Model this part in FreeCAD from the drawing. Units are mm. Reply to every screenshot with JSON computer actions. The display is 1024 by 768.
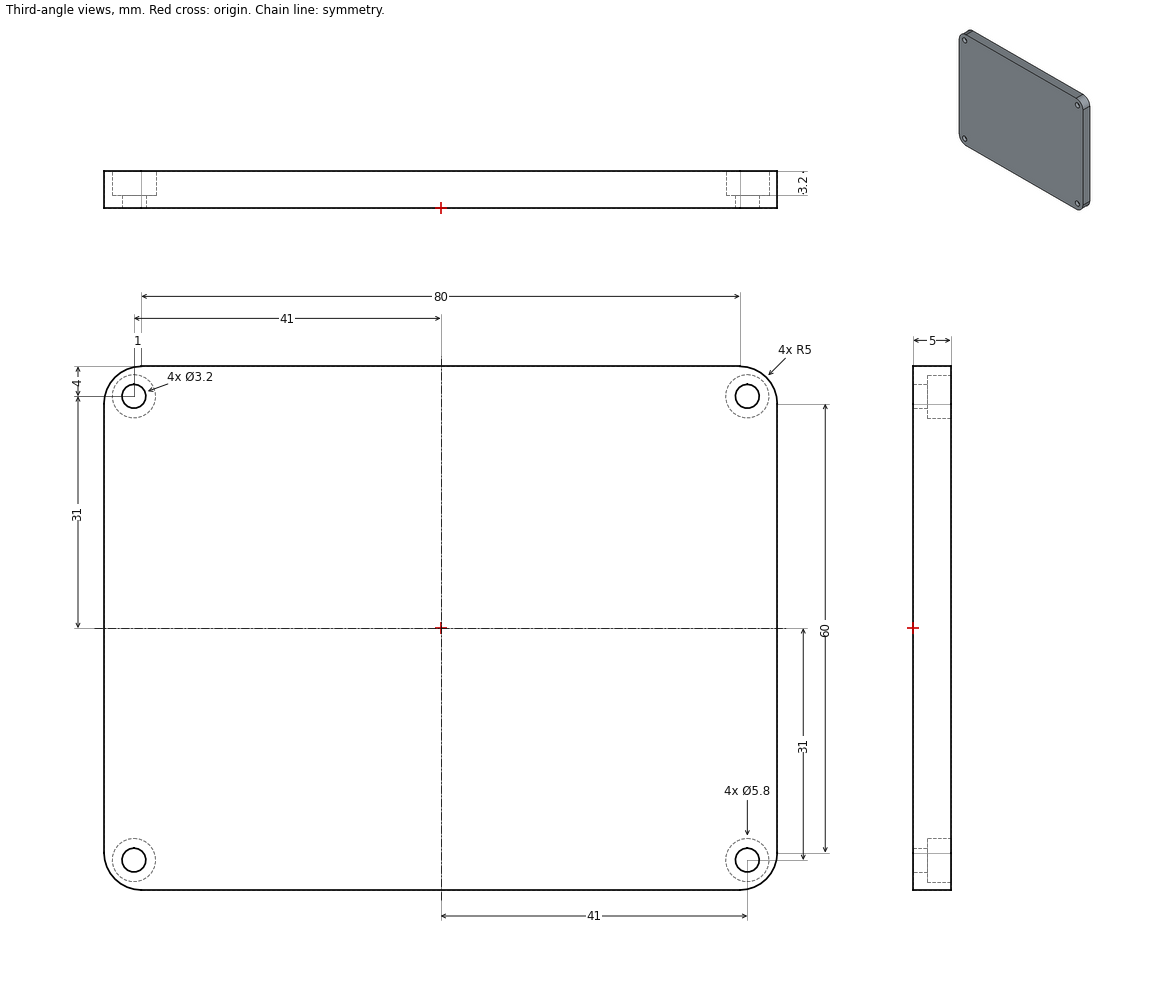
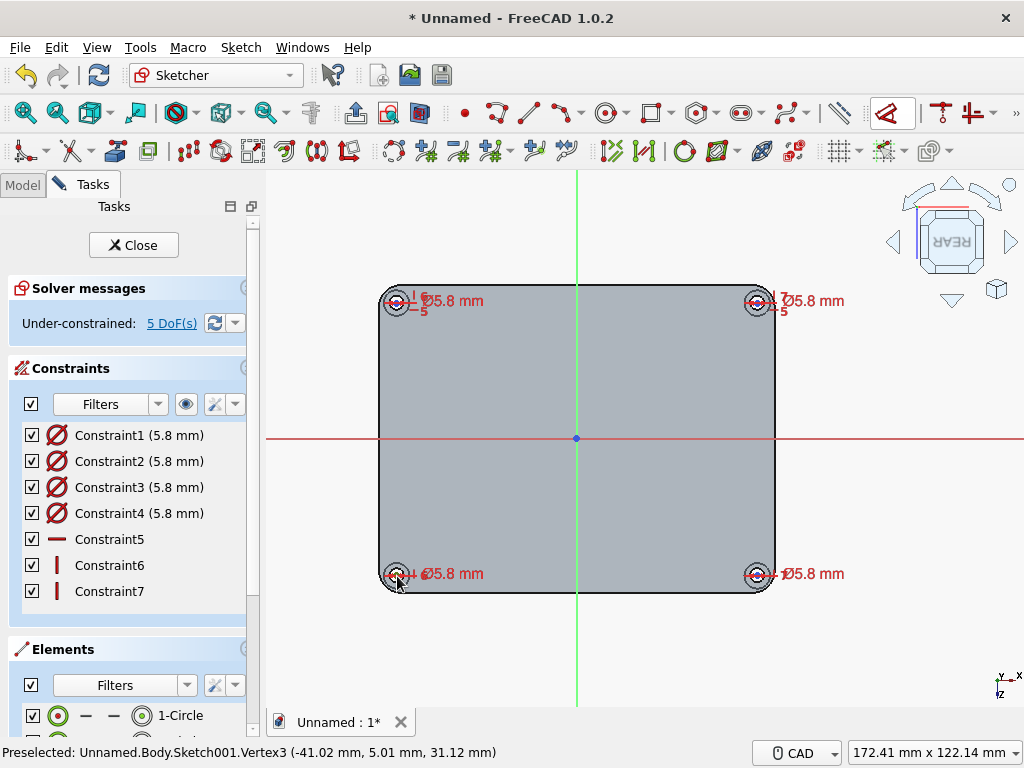
{"action": "left_click", "coordinate": [757, 576]}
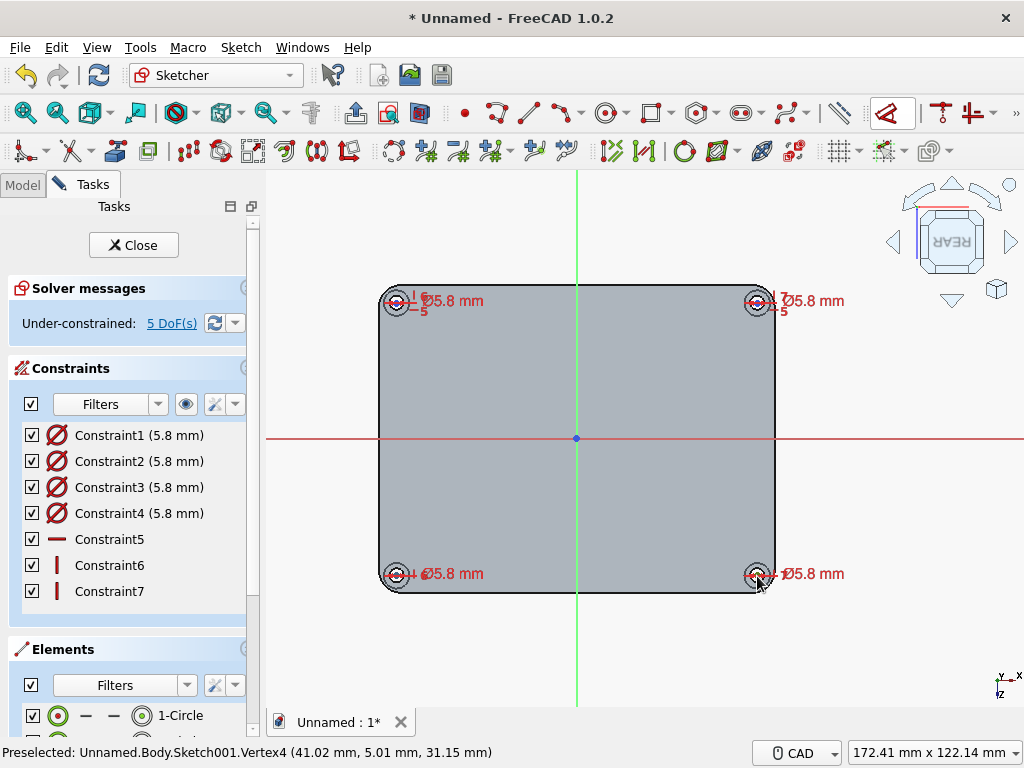
{"action": "key", "text": "h"}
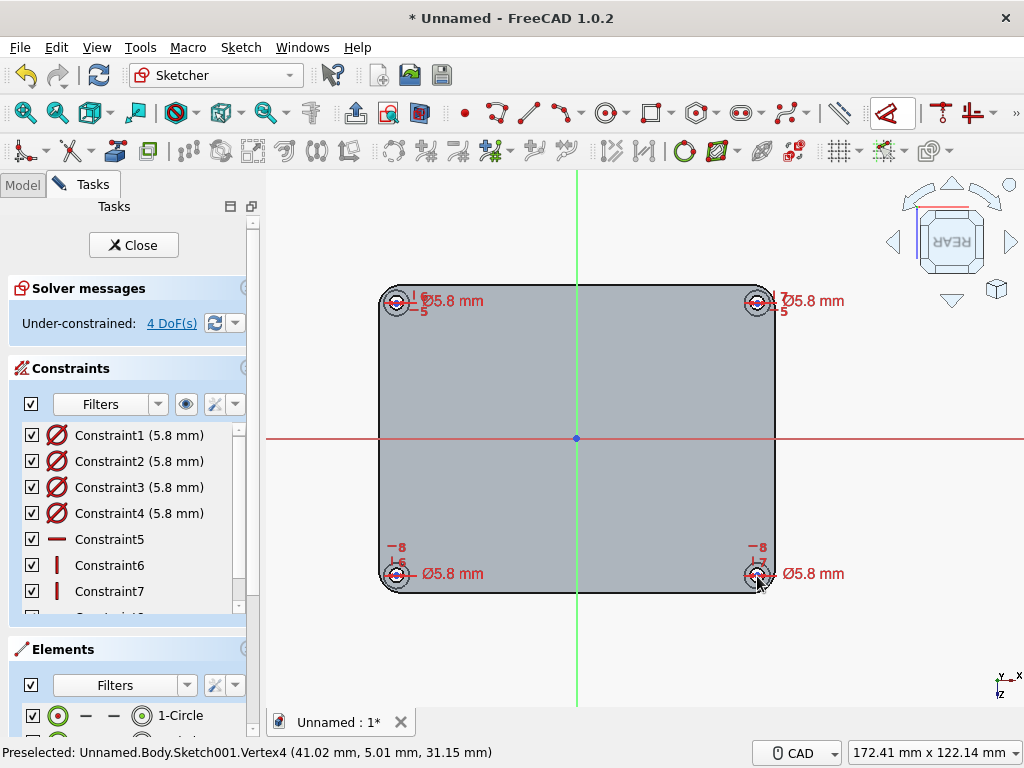
{"action": "left_click", "coordinate": [757, 303]}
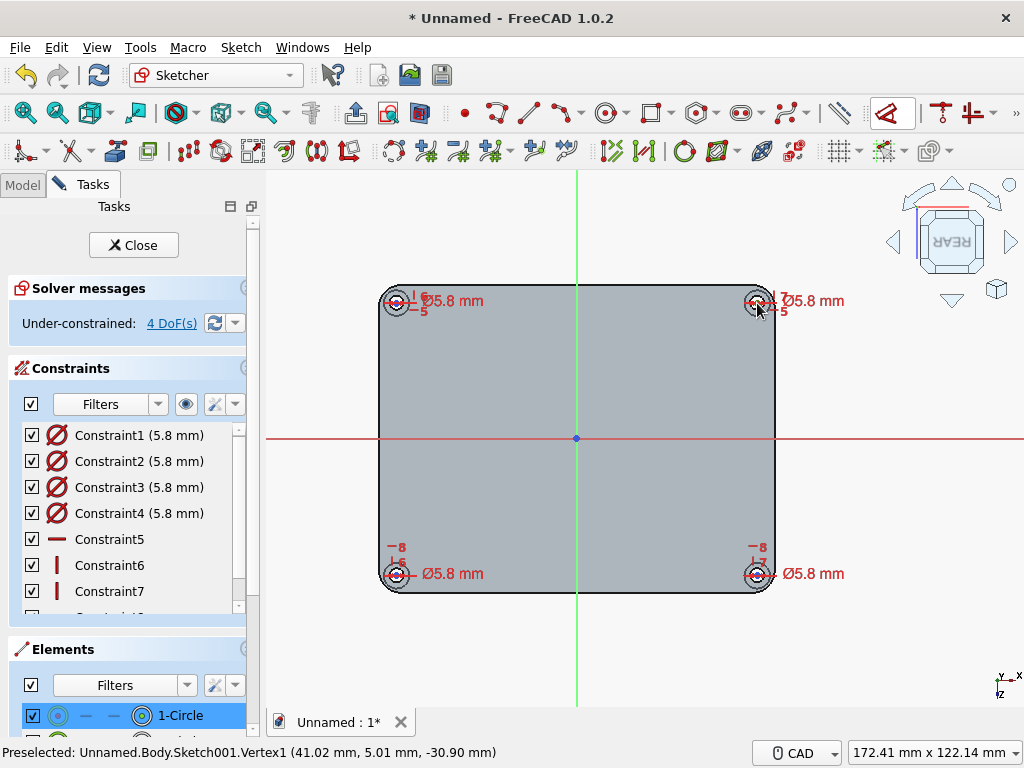
{"action": "left_click", "coordinate": [910, 114]}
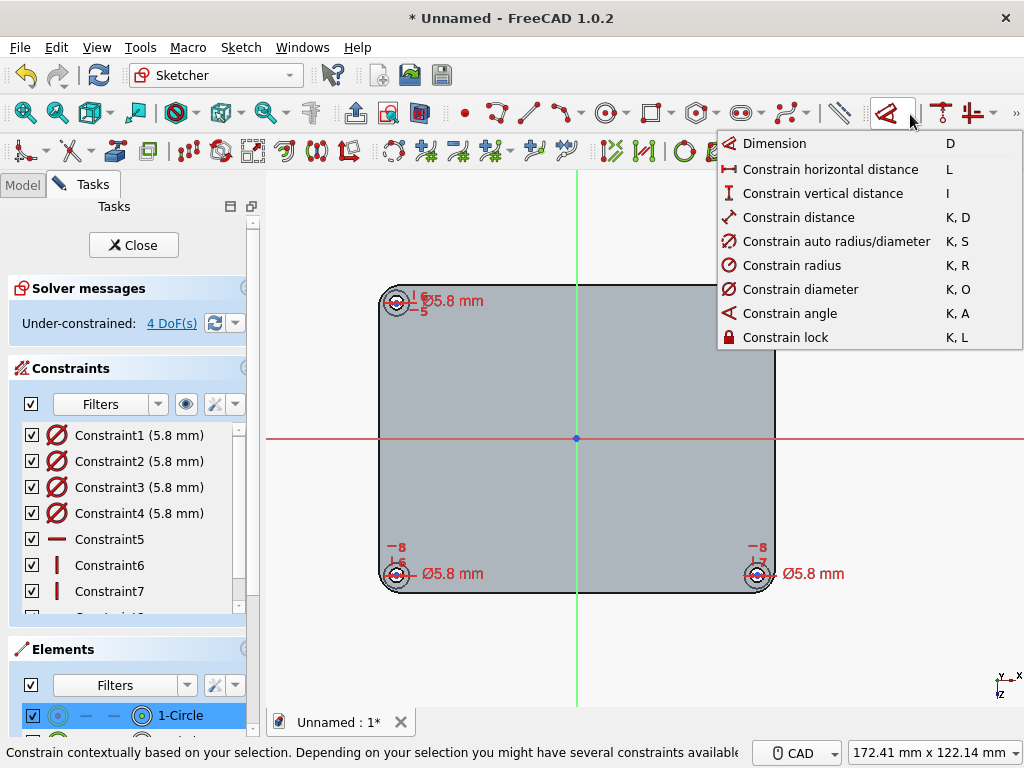
{"action": "left_click", "coordinate": [870, 169]}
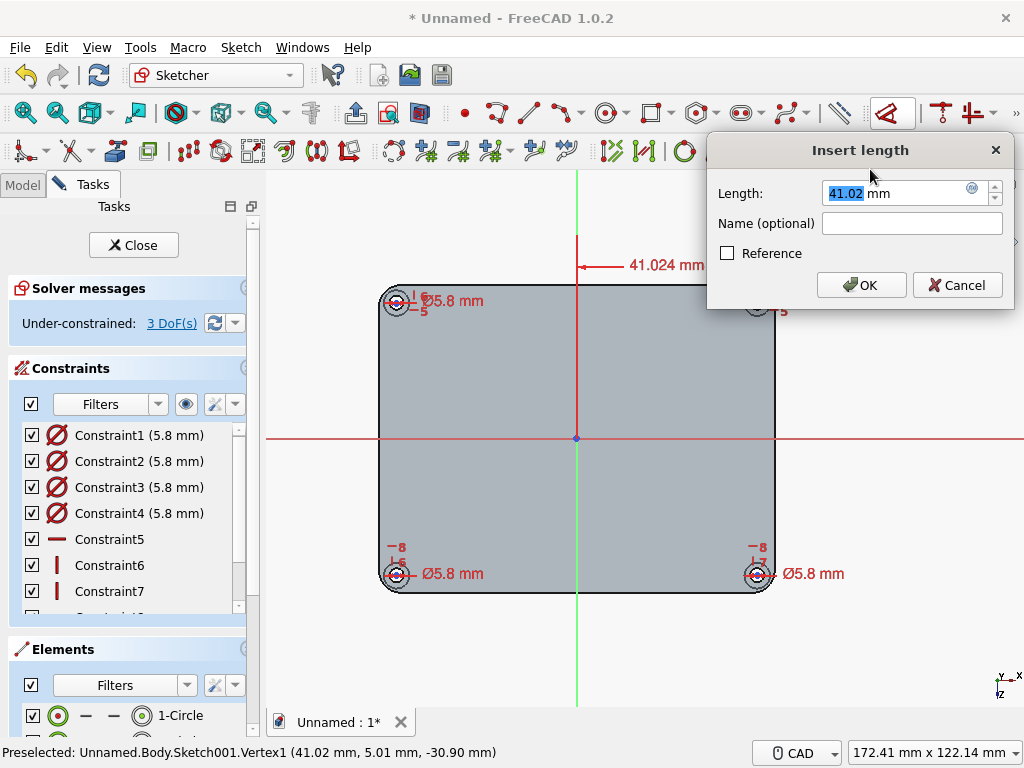
{"action": "type", "text": "41"}
{"action": "key", "text": "Return"}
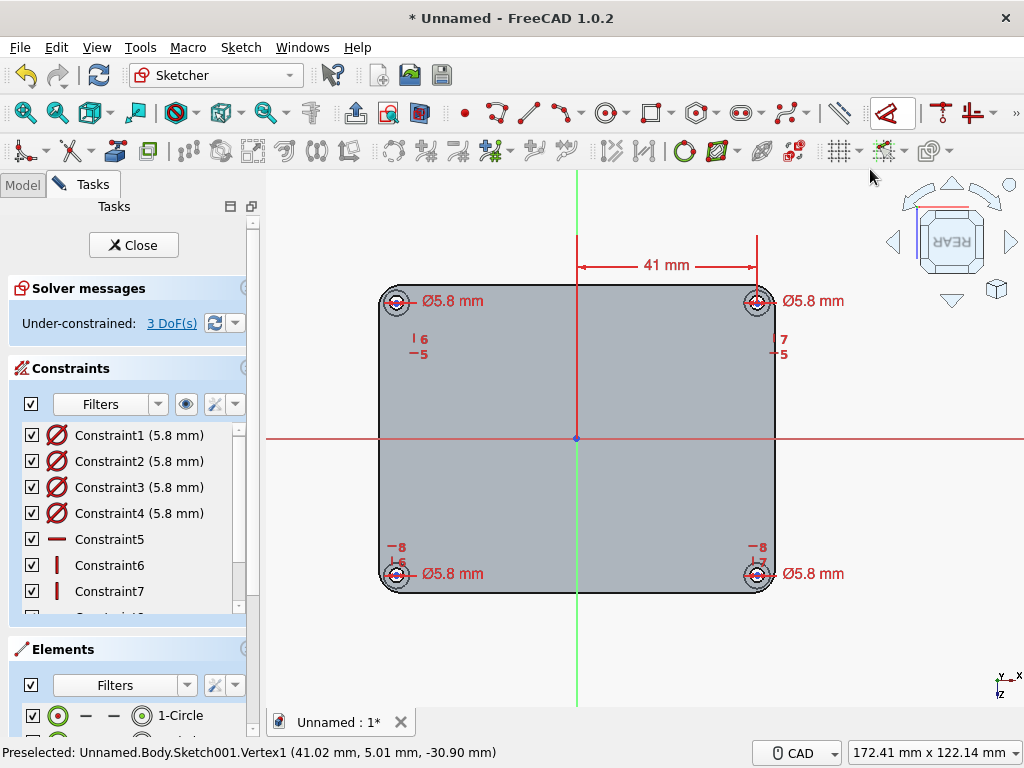
{"action": "left_click", "coordinate": [757, 303]}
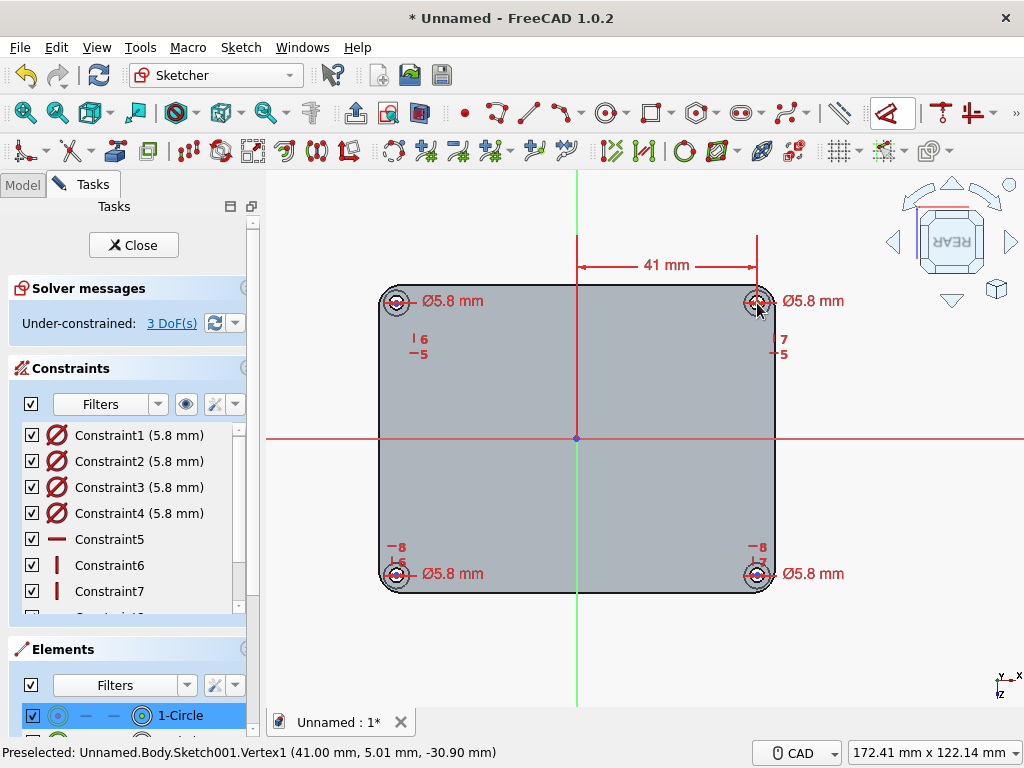
{"action": "key", "text": "i"}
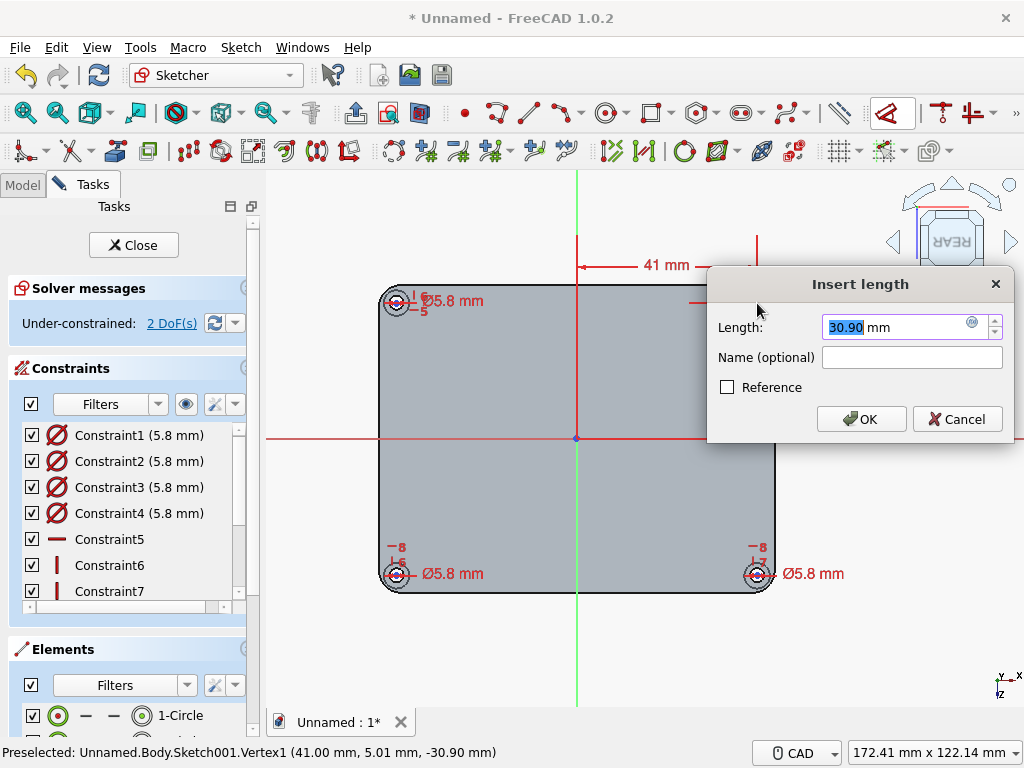
{"action": "type", "text": "31"}
{"action": "key", "text": "Return"}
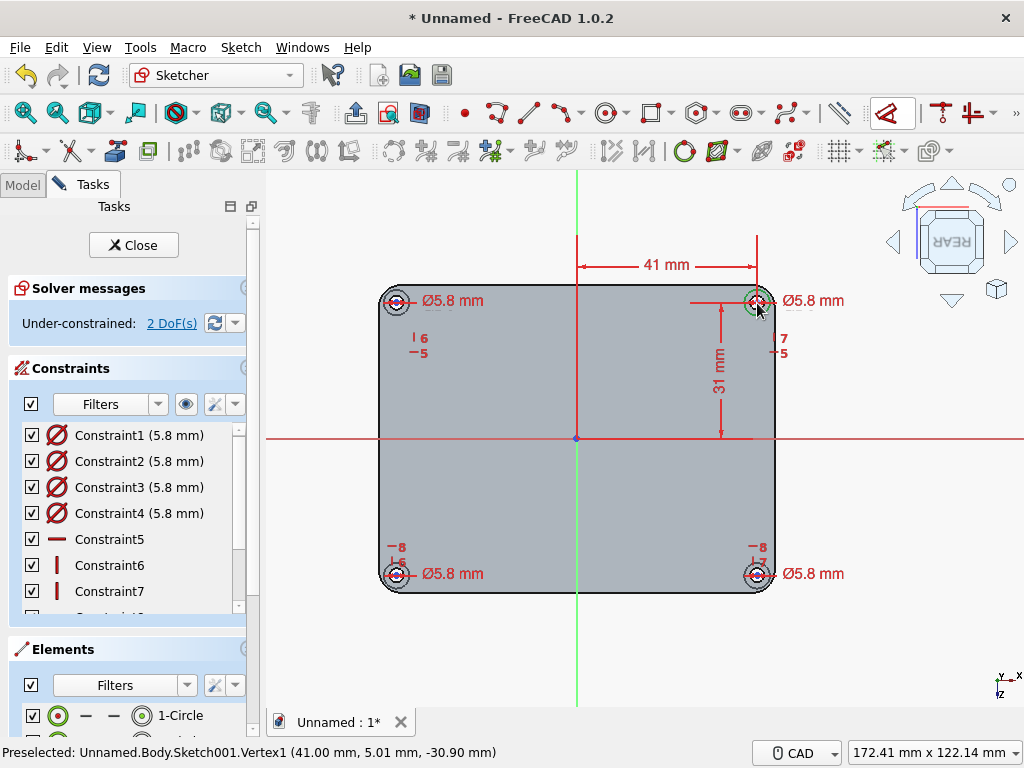
{"action": "left_click", "coordinate": [397, 303]}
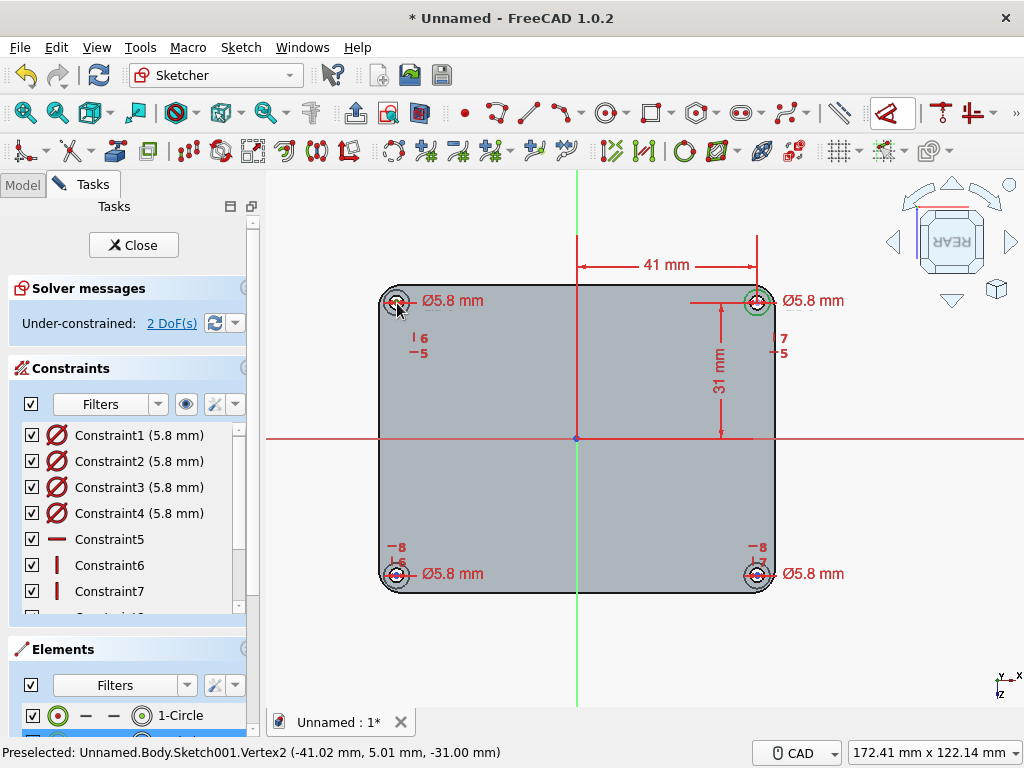
{"action": "key", "text": "l"}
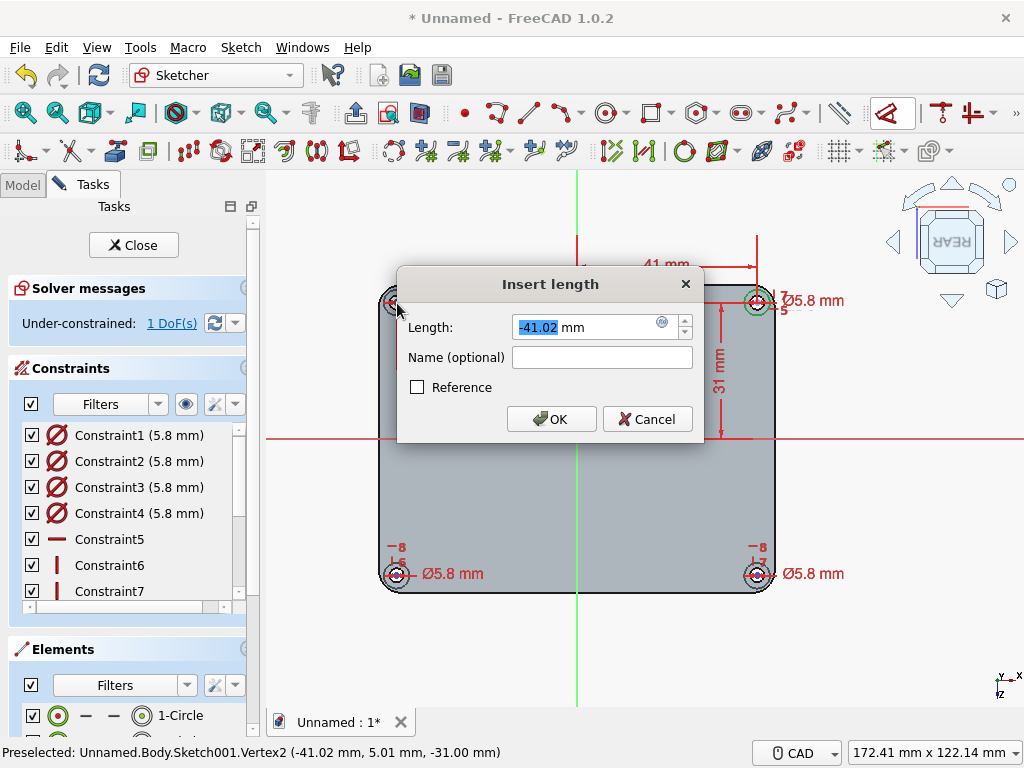
{"action": "type", "text": "-41"}
{"action": "key", "text": "Return"}